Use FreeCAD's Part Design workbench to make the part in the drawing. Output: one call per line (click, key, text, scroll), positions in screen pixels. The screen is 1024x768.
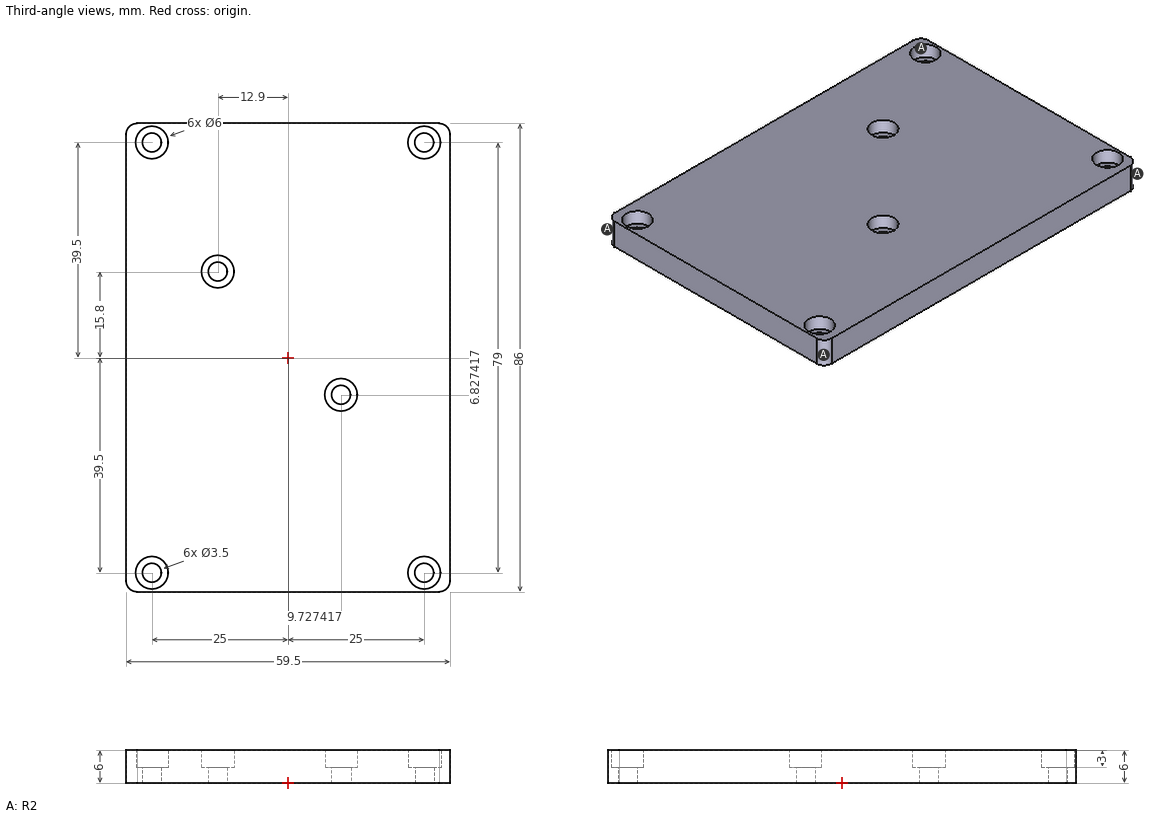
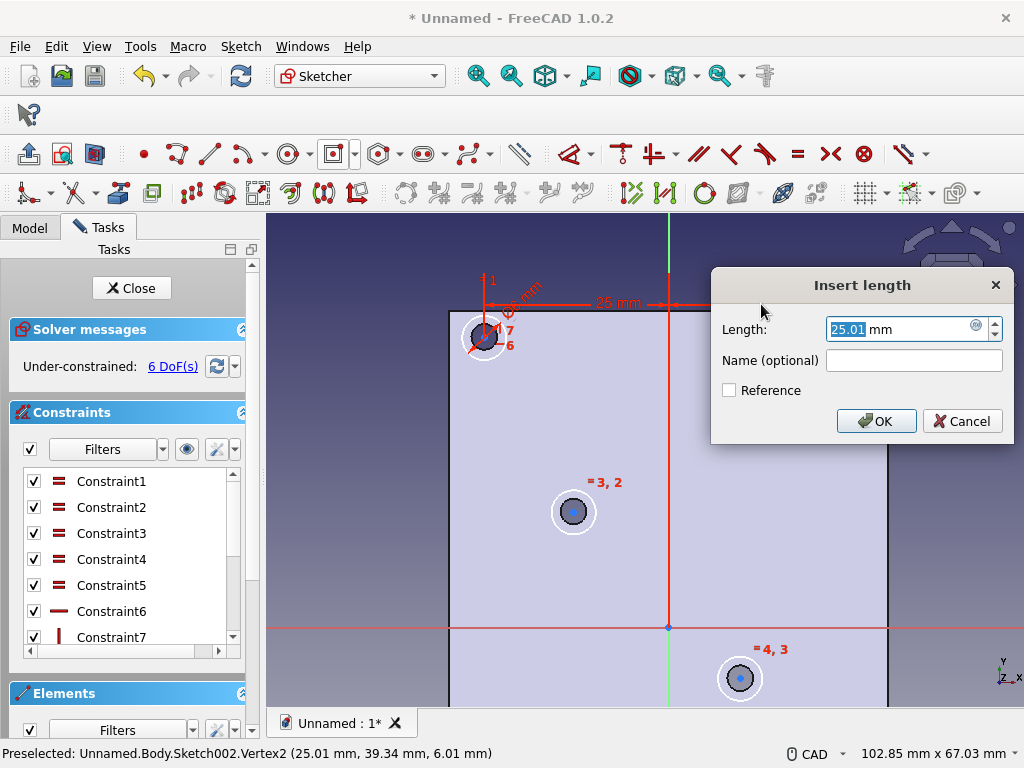
text(25)
key(Return)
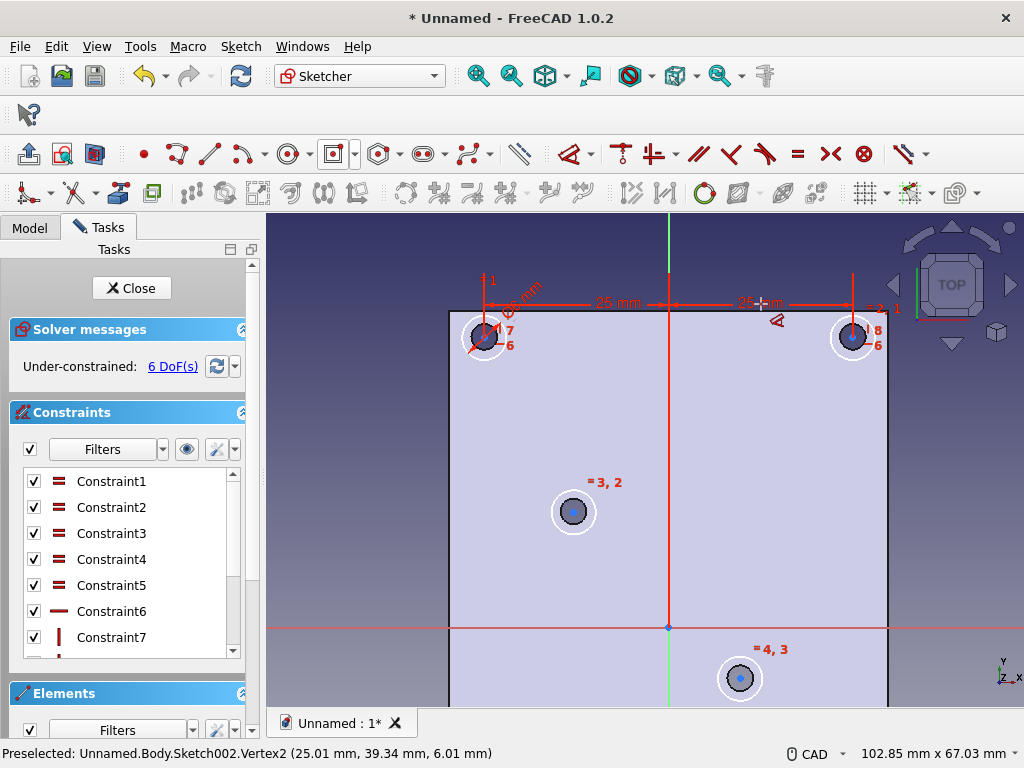
click(484, 338)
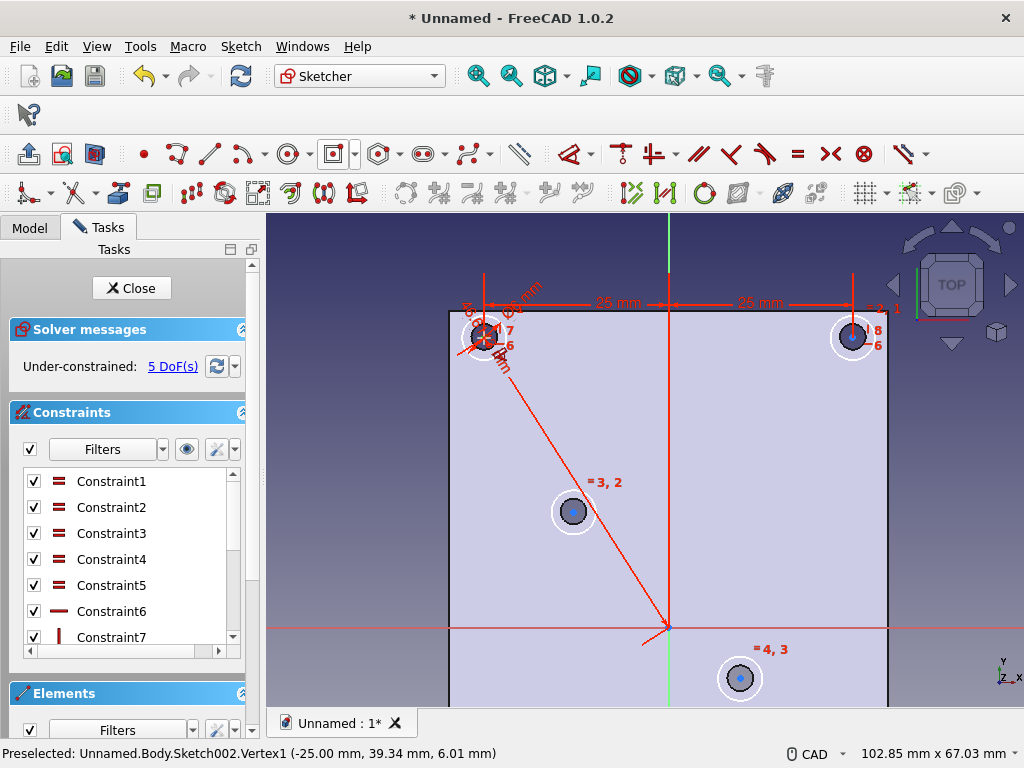
scroll(501, 323, down, 4)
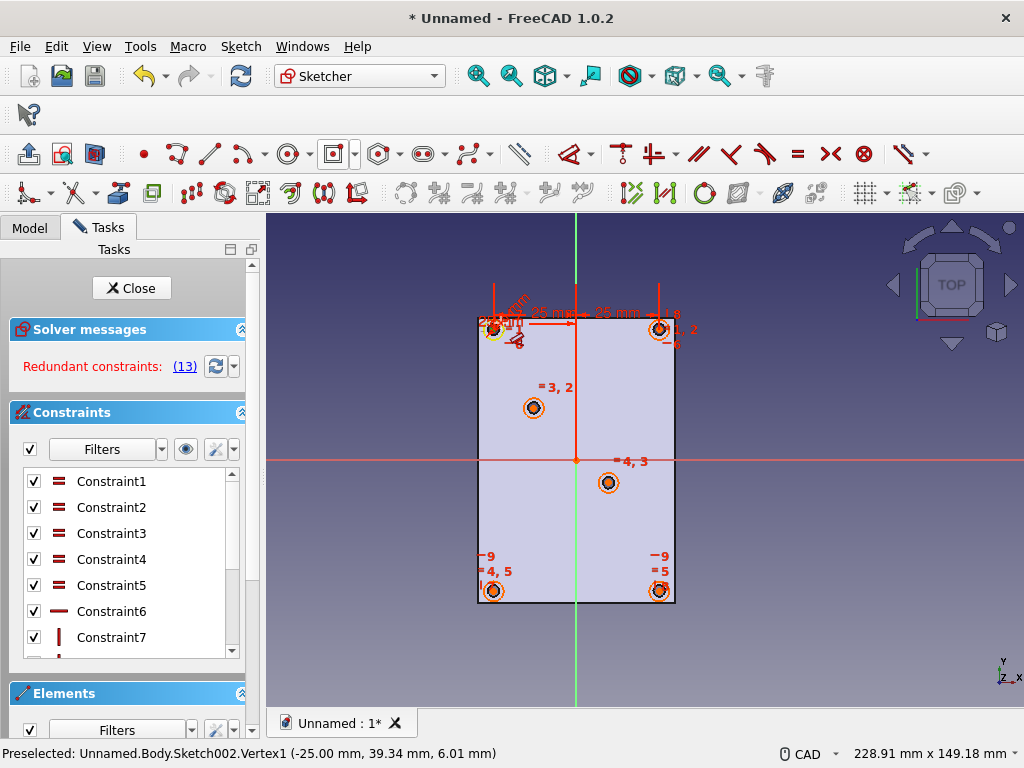
click(494, 591)
click(460, 400)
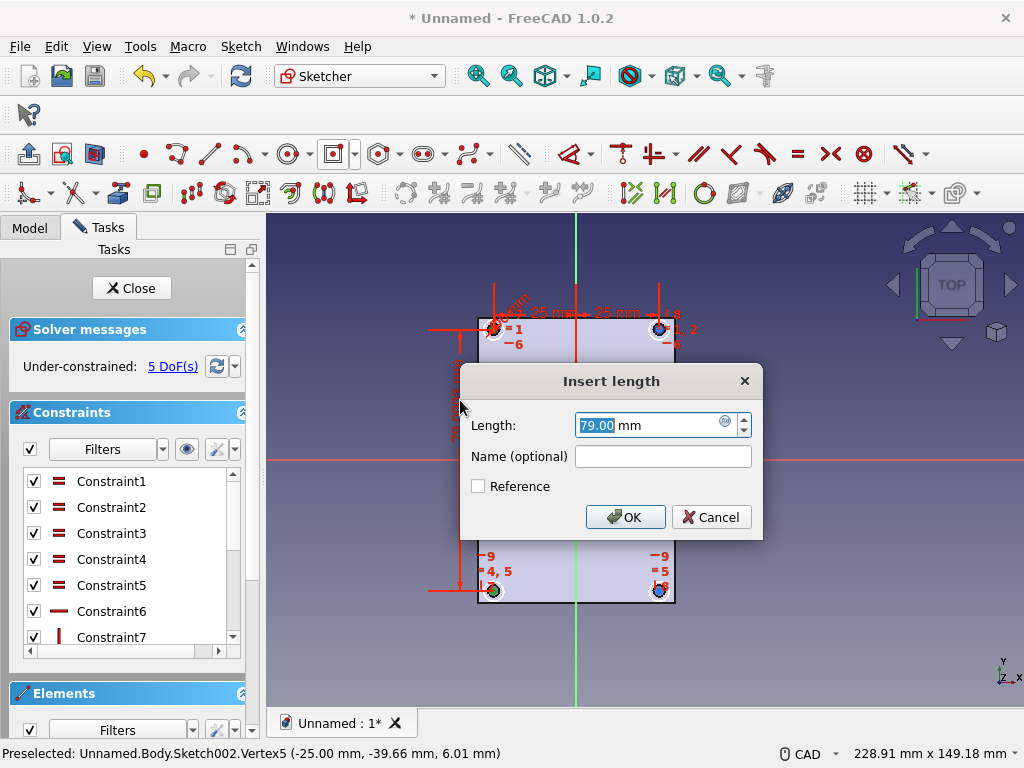
text(79)
key(Return)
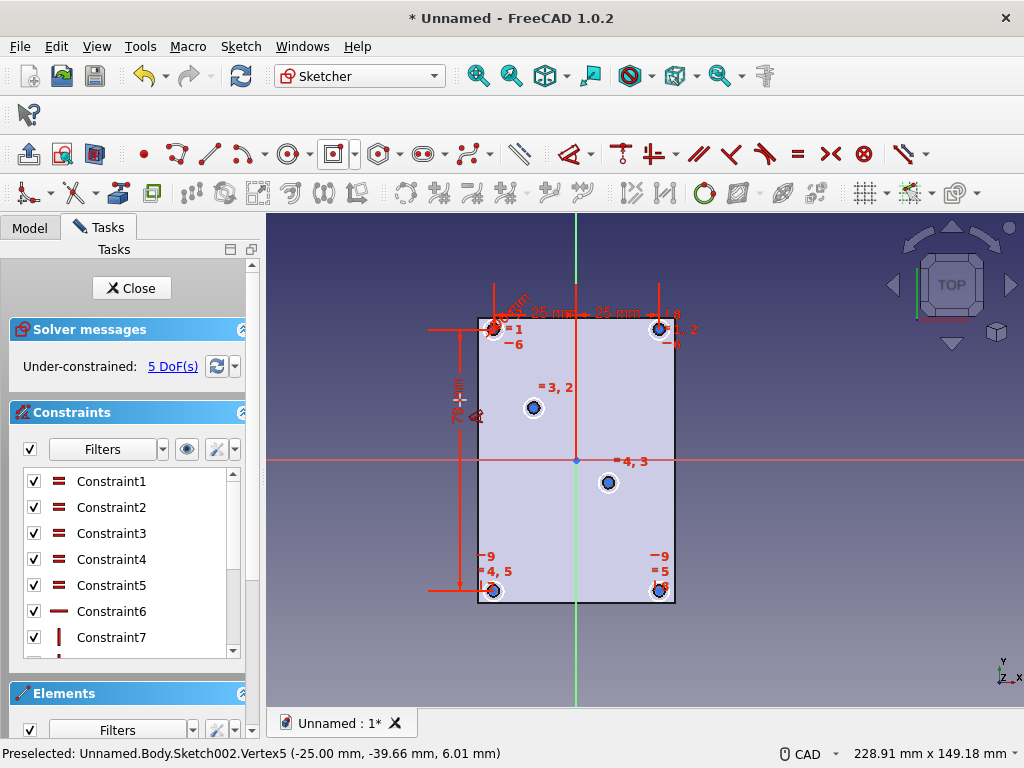
click(494, 330)
click(460, 365)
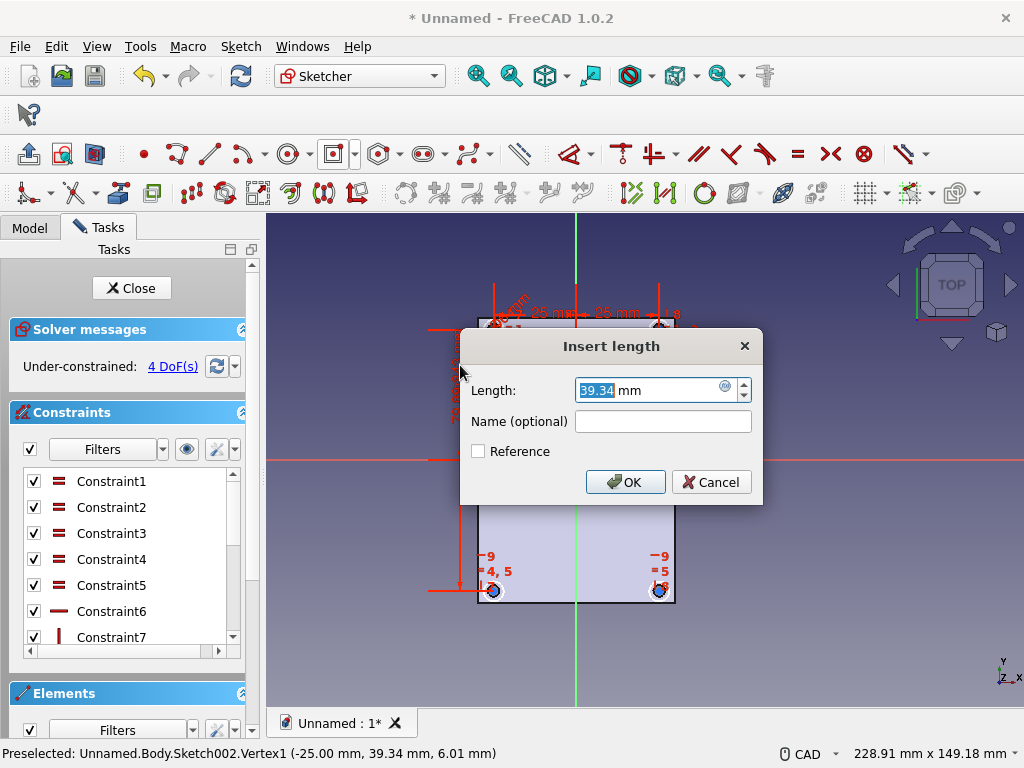
text(39.5)
key(Return)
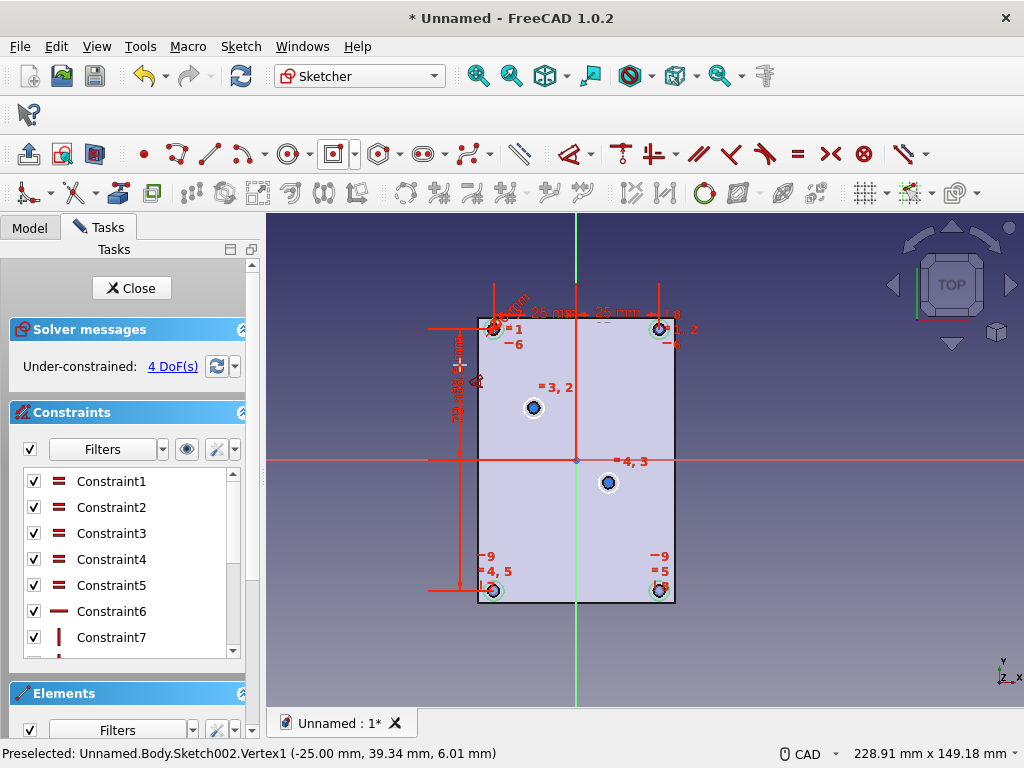
click(534, 408)
click(555, 374)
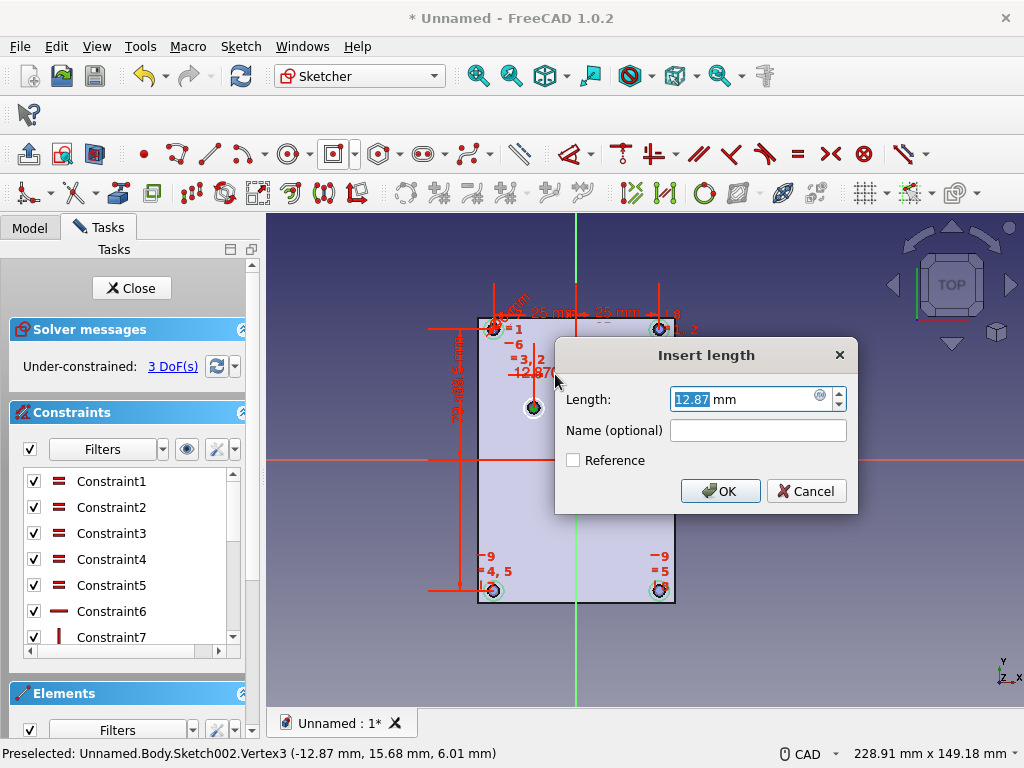
text(12.9)
key(Return)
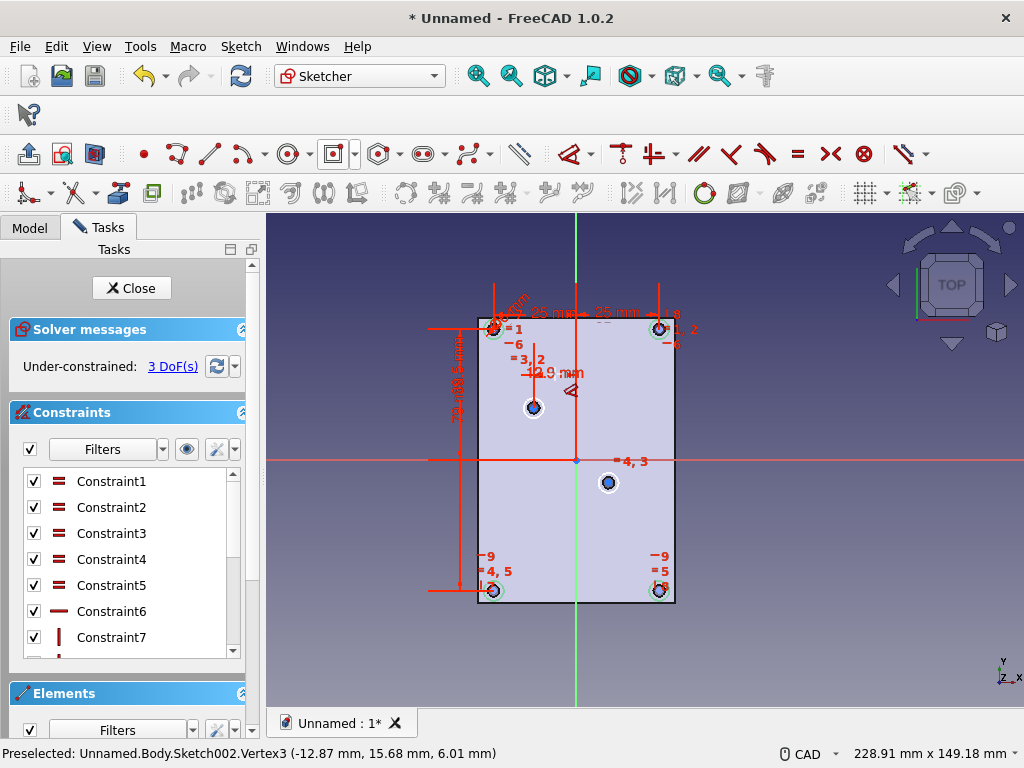
click(534, 408)
click(500, 434)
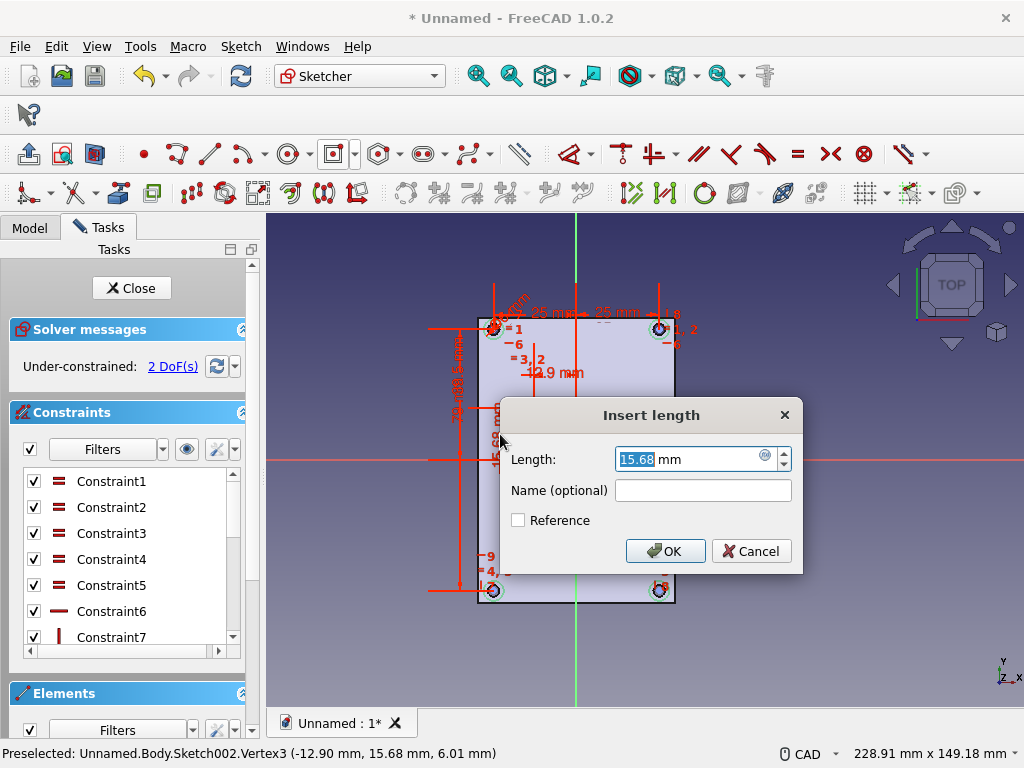
text(15.8)
key(Return)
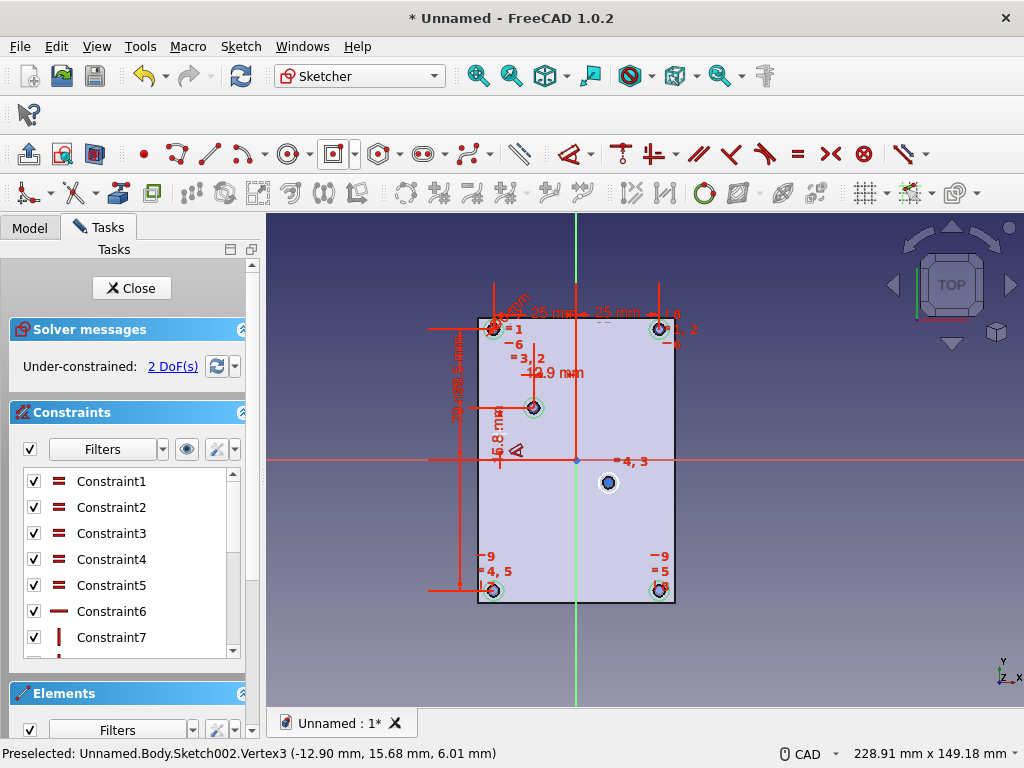
scroll(609, 483, up, 2)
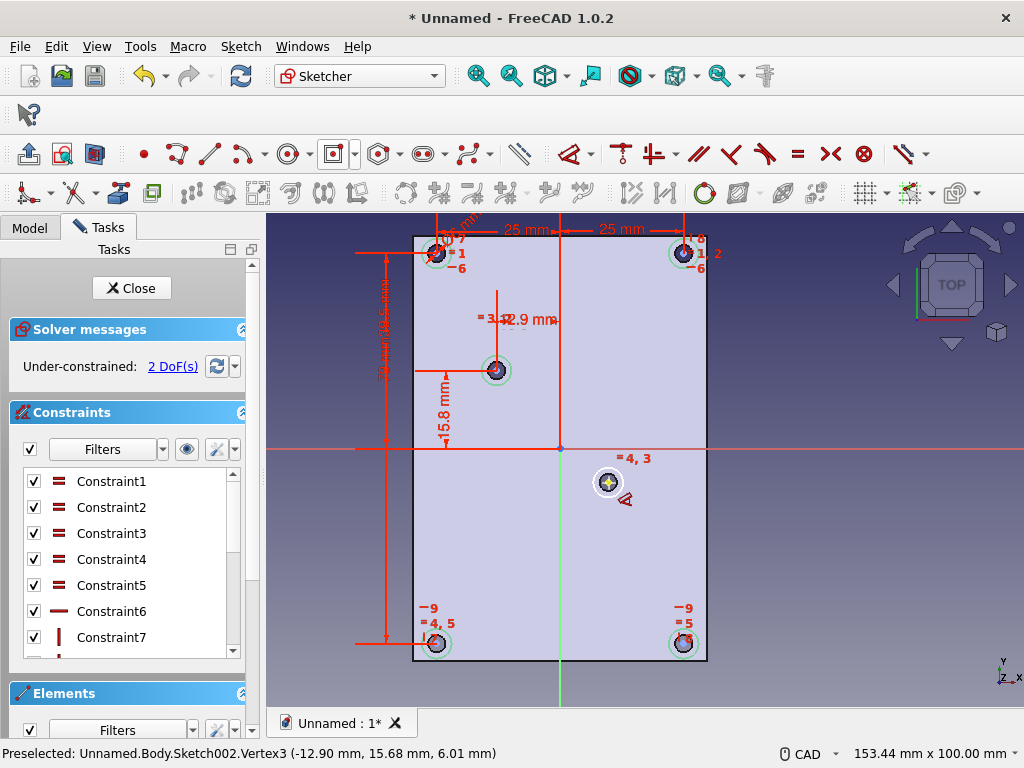
click(608, 483)
click(584, 517)